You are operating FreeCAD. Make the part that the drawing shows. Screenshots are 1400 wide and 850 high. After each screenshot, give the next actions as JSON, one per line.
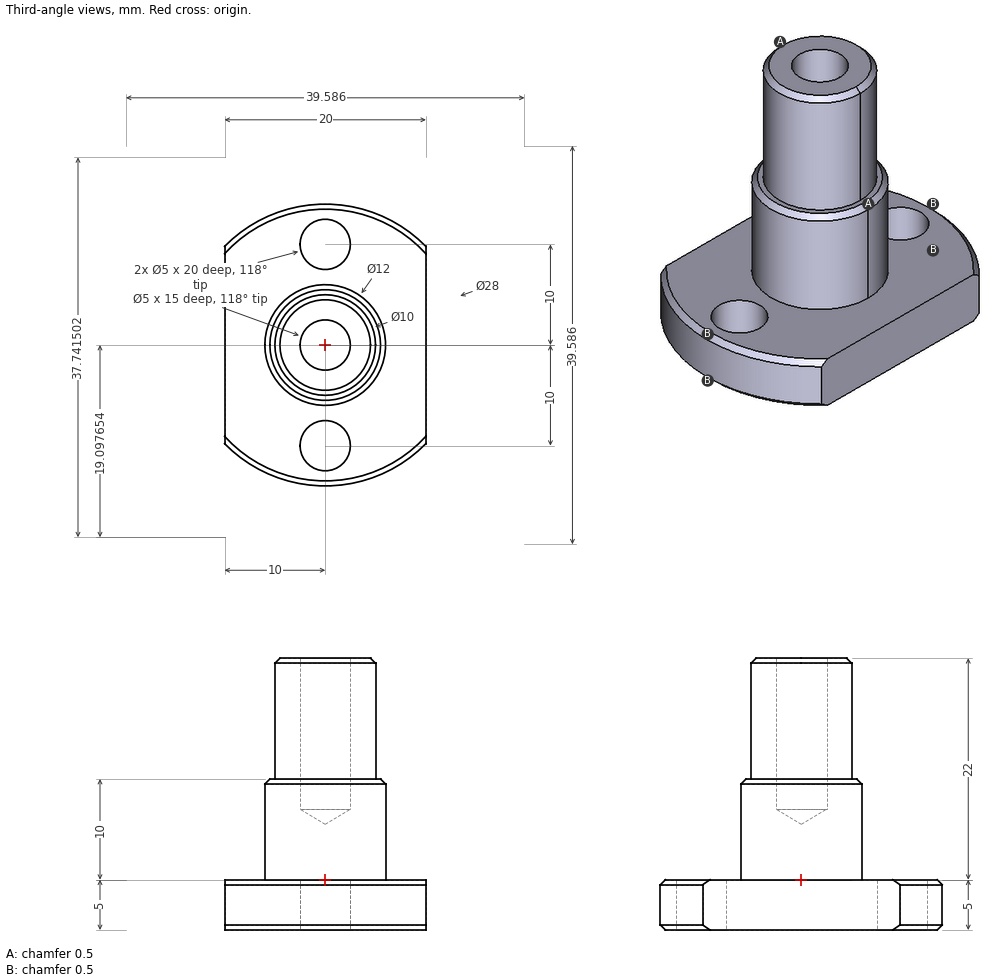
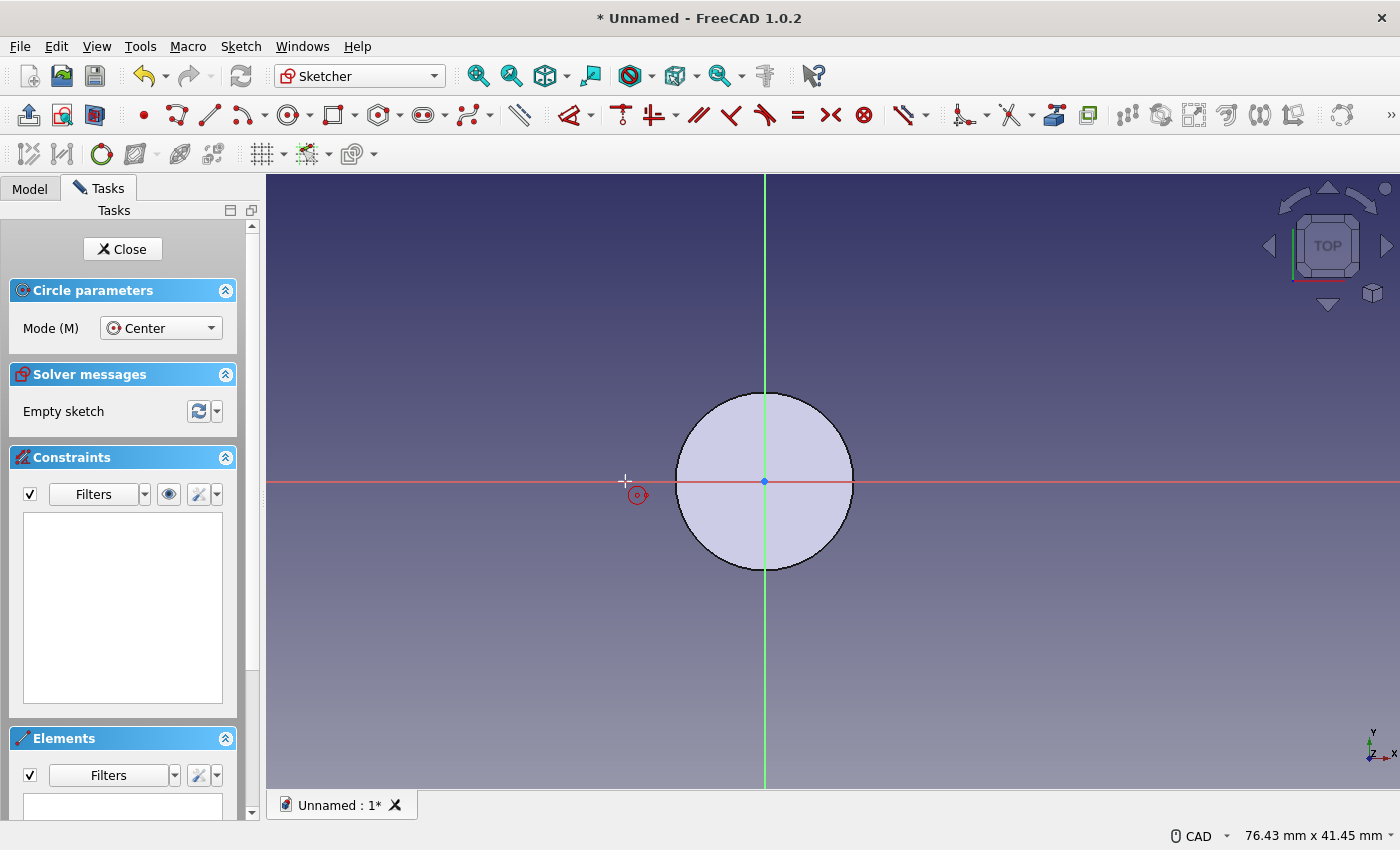
{"action": "left_click", "coordinate": [765, 482]}
{"action": "mouse_move", "coordinate": [911, 335]}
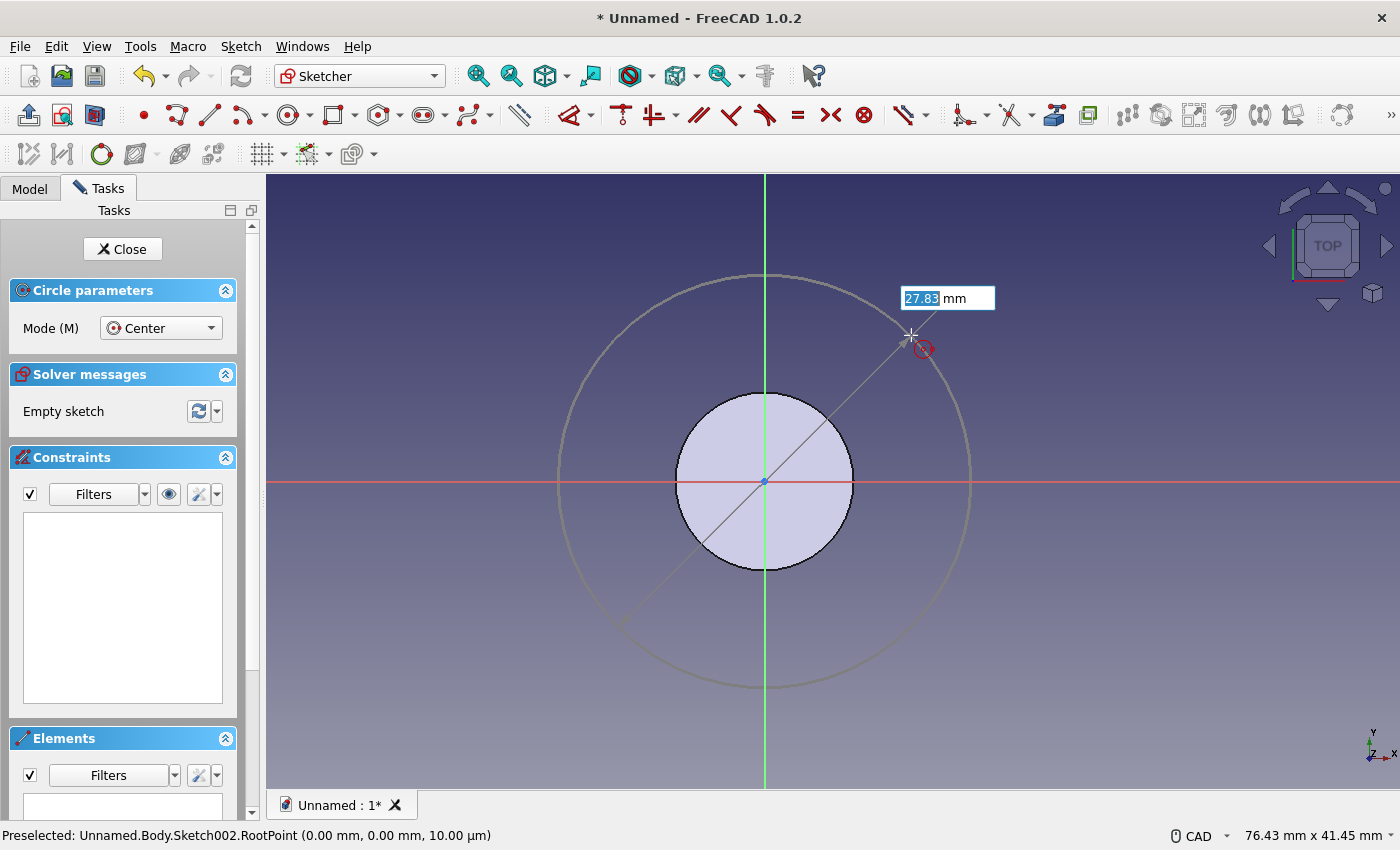
{"action": "type", "text": "28"}
{"action": "key", "text": "Return"}
{"action": "key", "text": "Escape"}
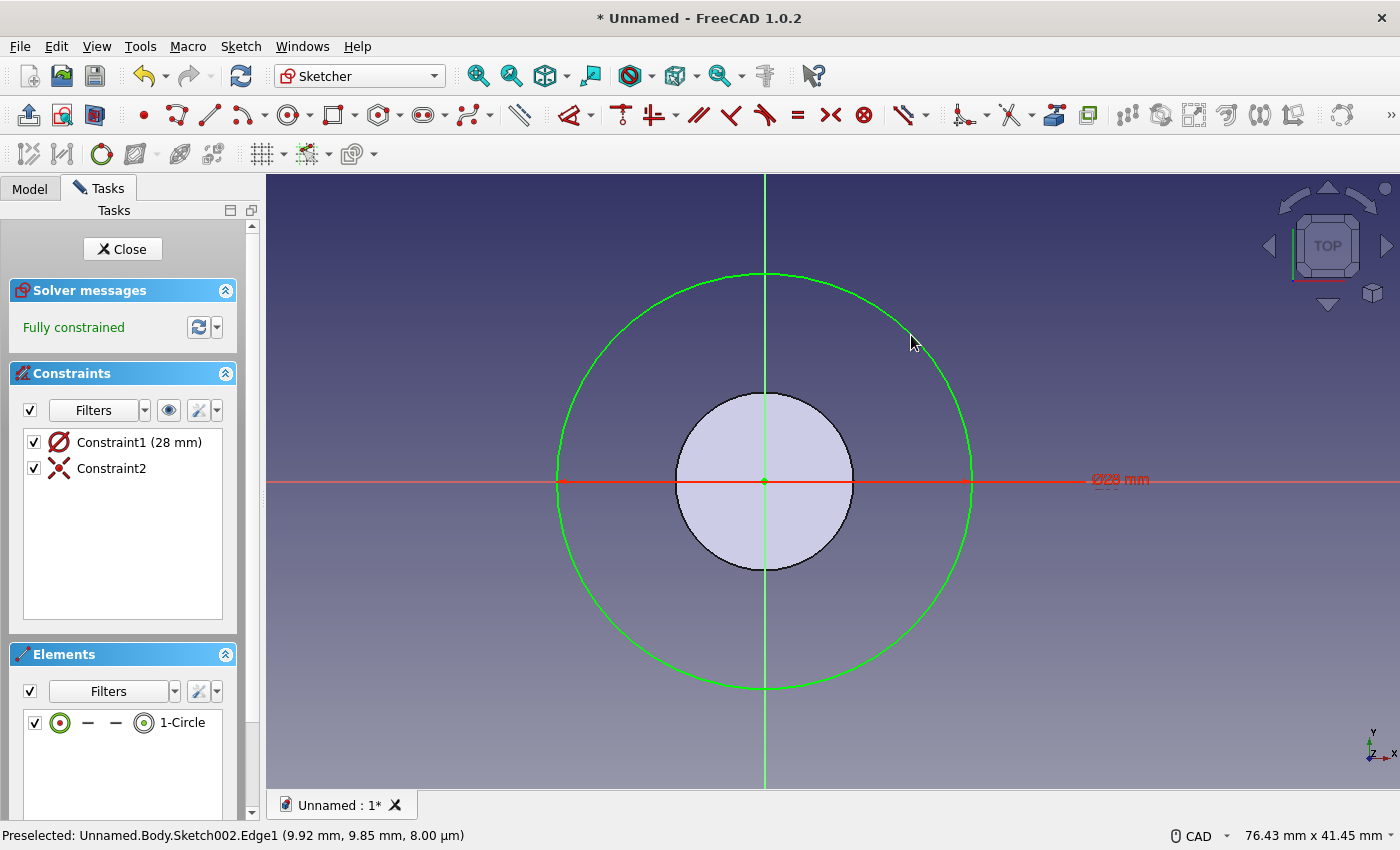
{"action": "left_click", "coordinate": [123, 249]}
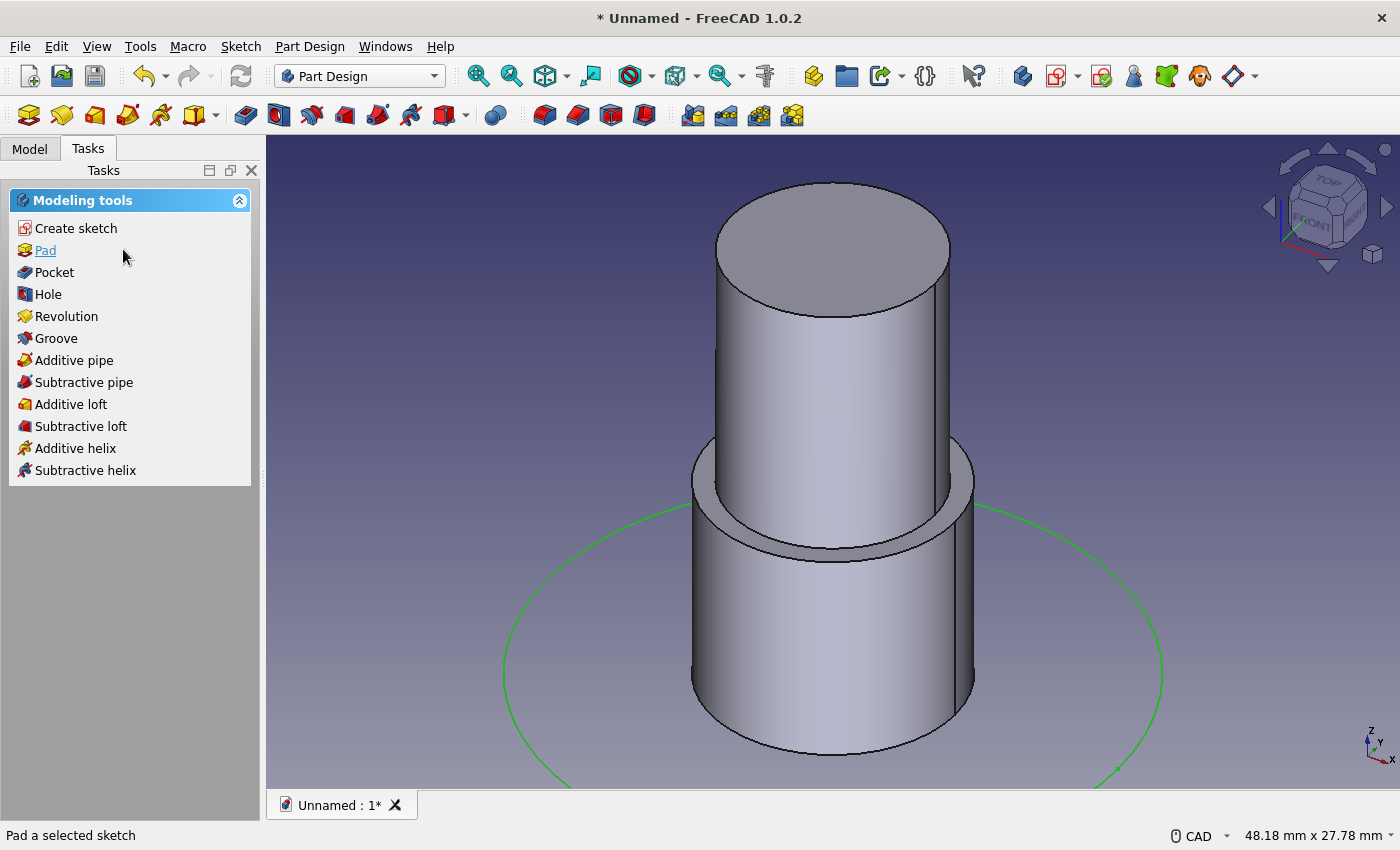
{"action": "left_click", "coordinate": [29, 116]}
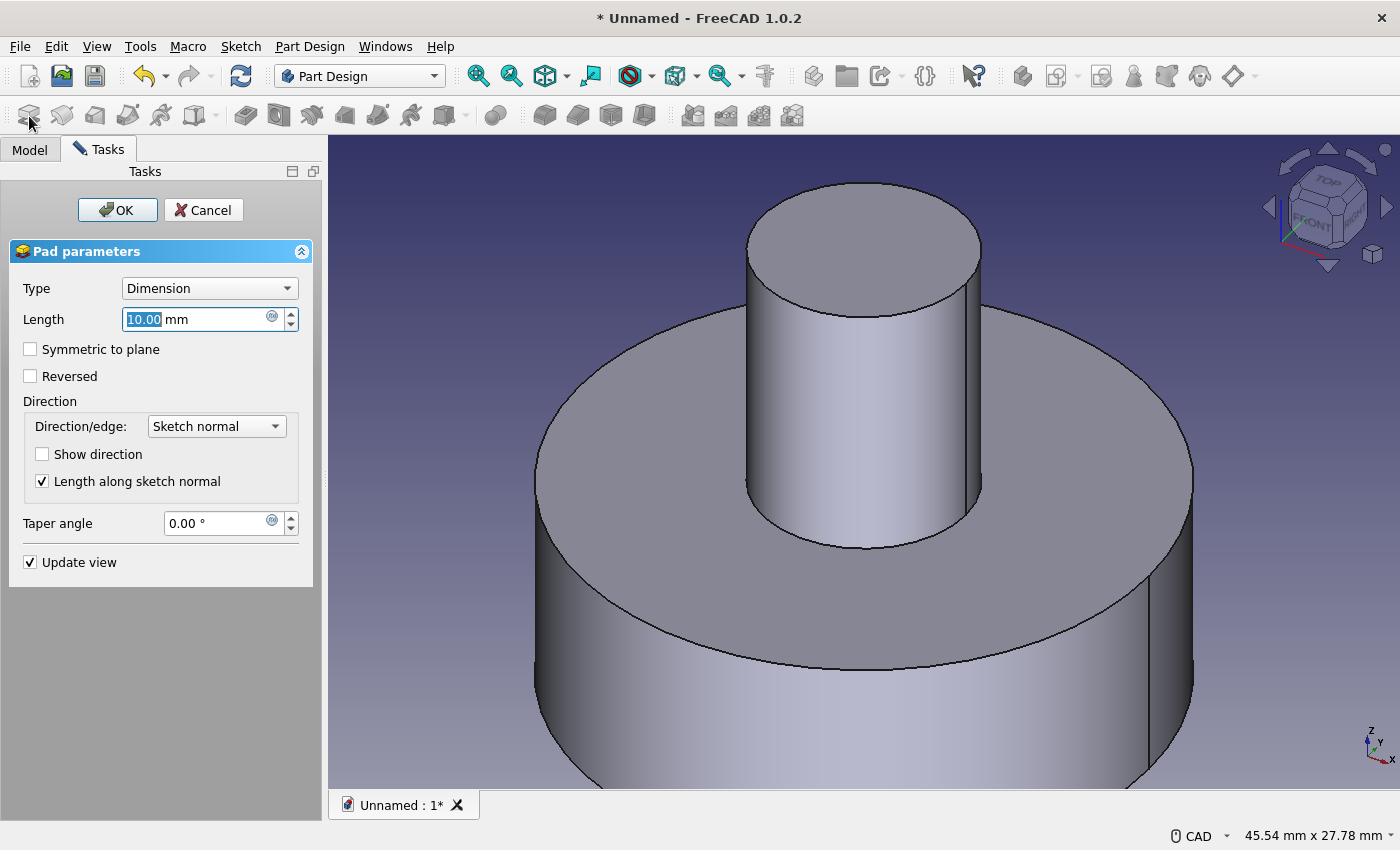
{"action": "type", "text": "5"}
{"action": "key", "text": "Tab"}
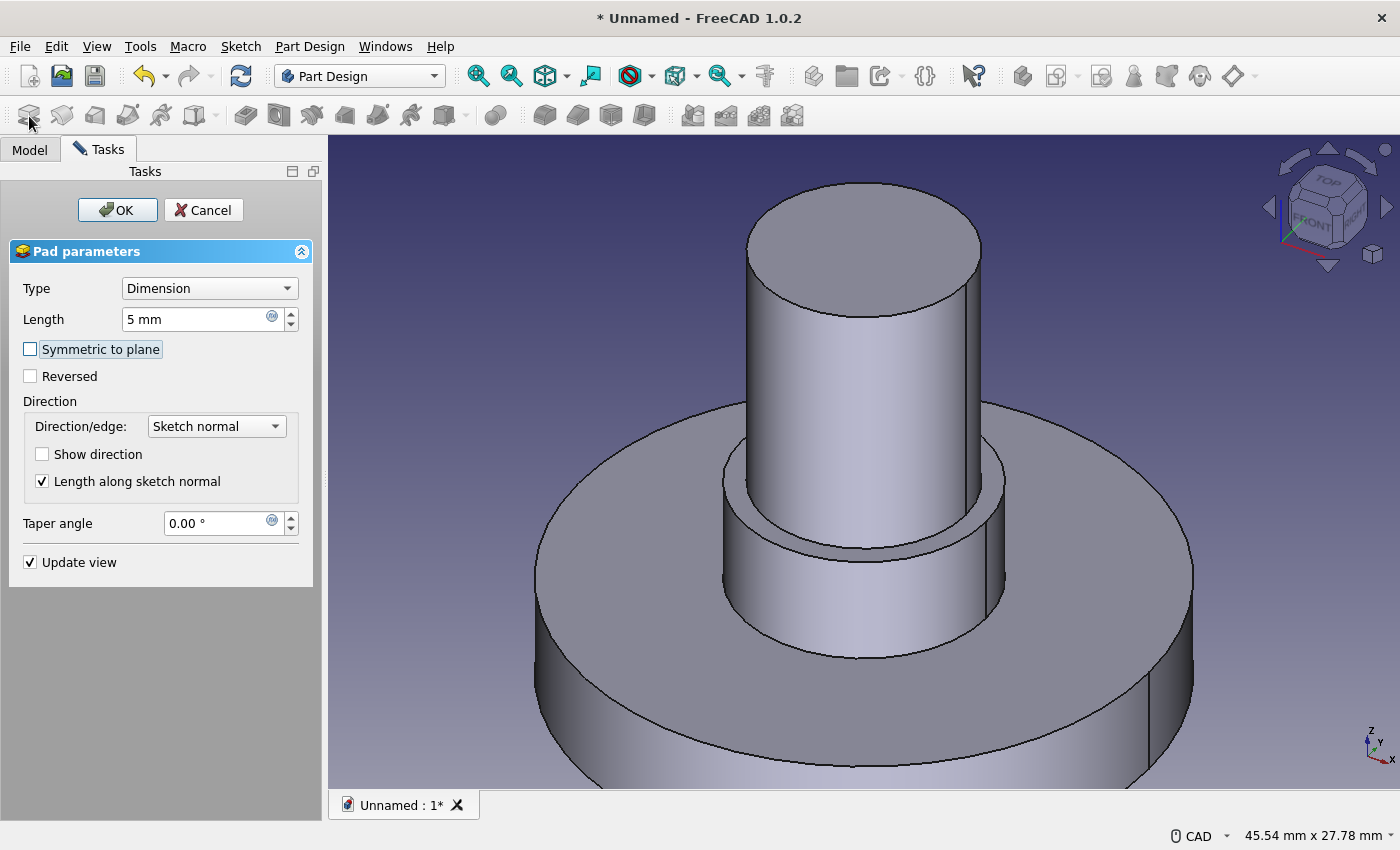
{"action": "left_click", "coordinate": [31, 376]}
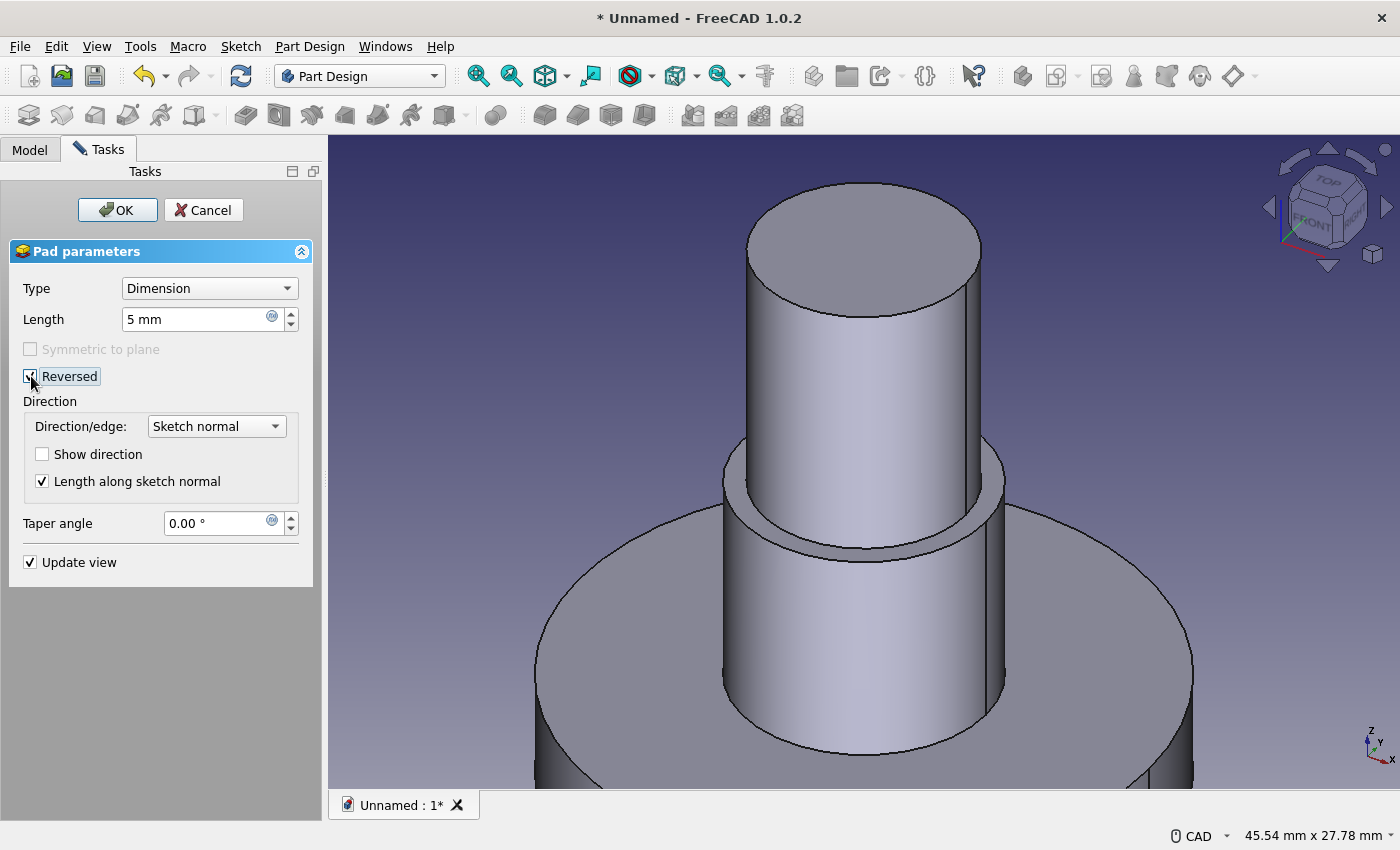
{"action": "left_click", "coordinate": [118, 210]}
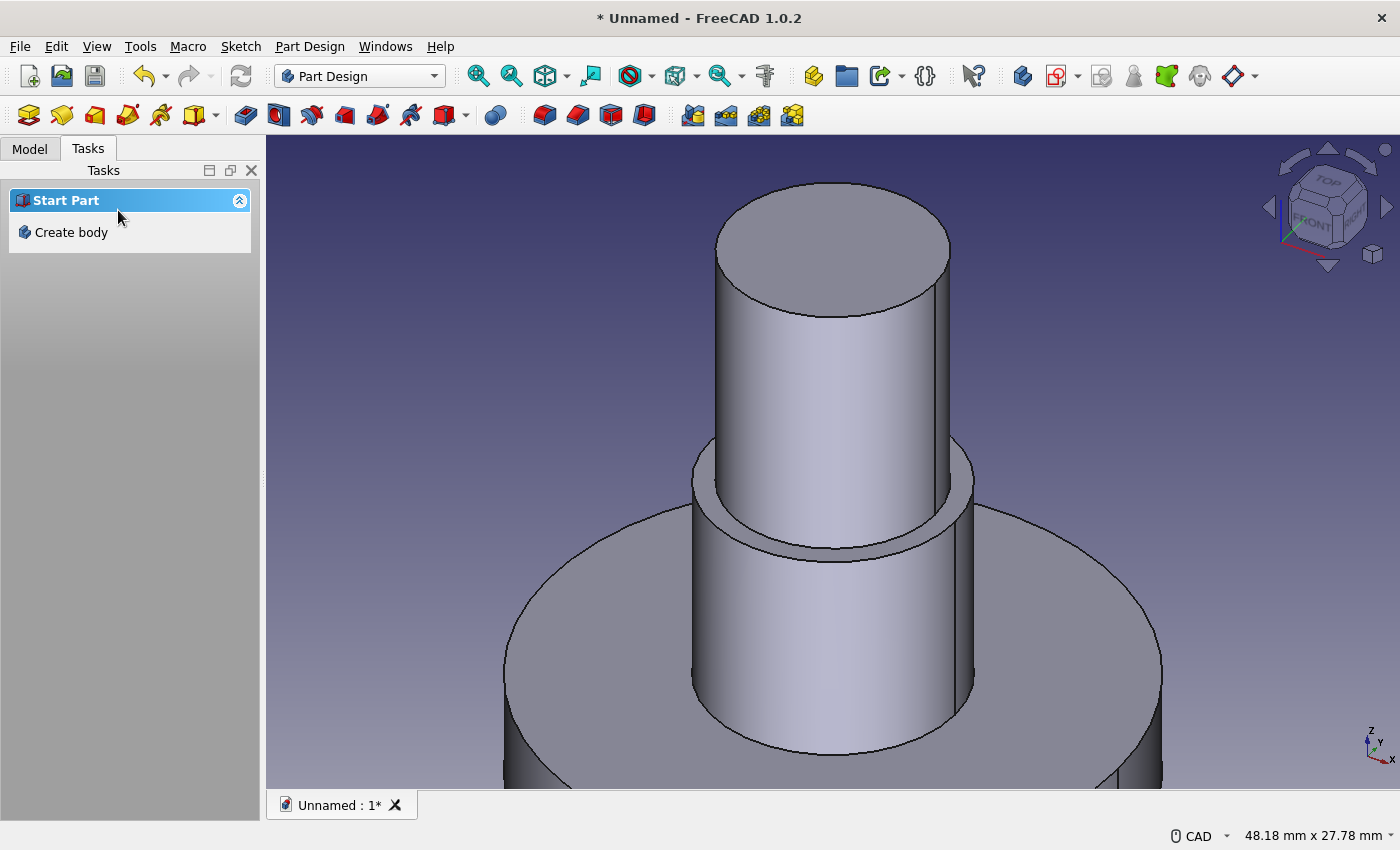
{"action": "key", "text": "v f"}